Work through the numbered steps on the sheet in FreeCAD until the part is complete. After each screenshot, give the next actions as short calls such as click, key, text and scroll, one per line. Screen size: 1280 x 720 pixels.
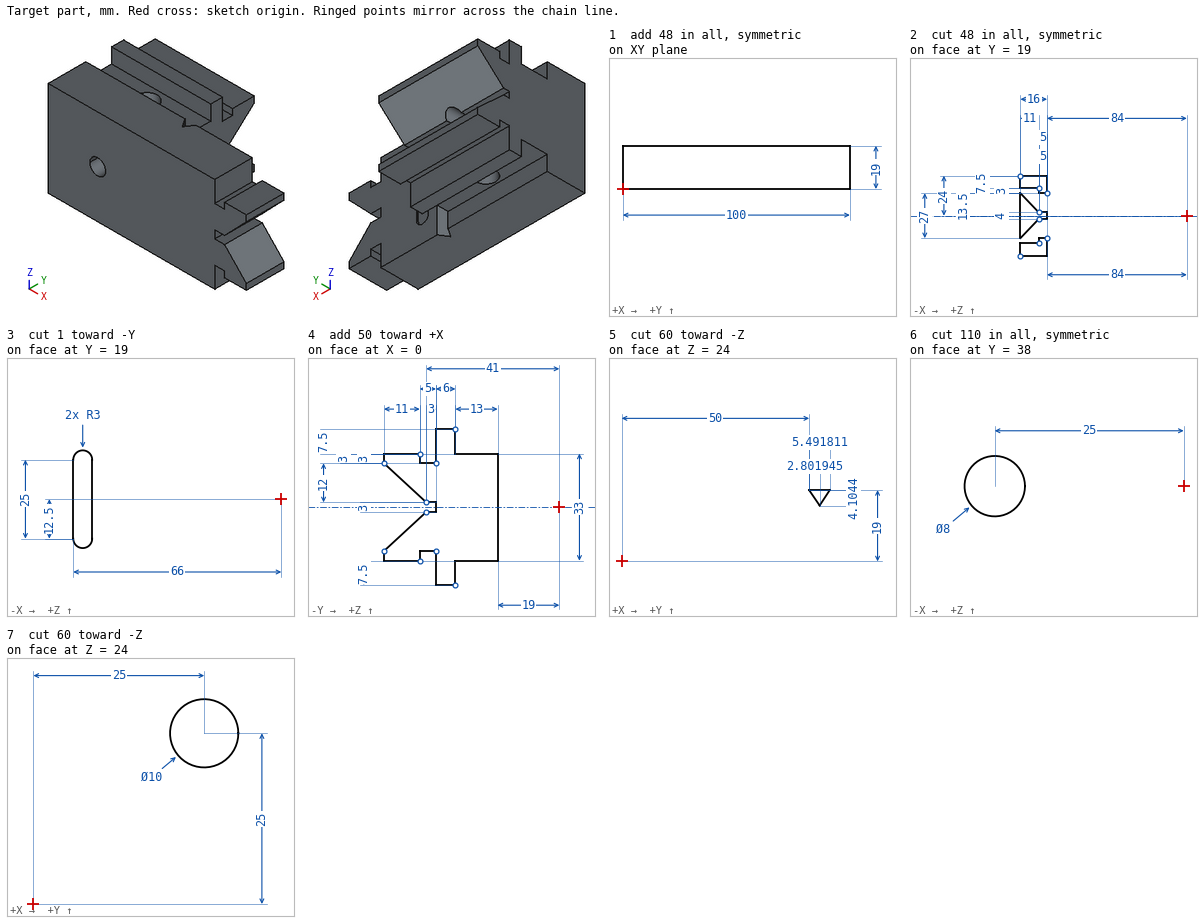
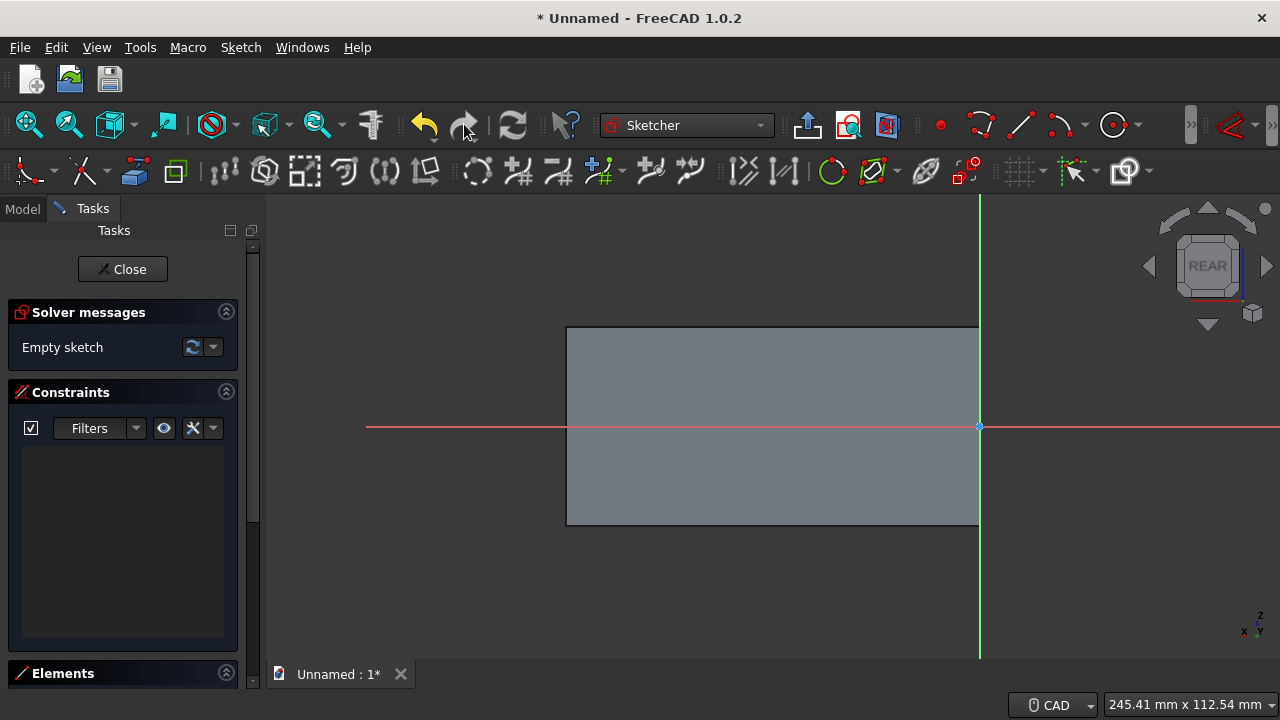
scroll(912, 426, up, 2)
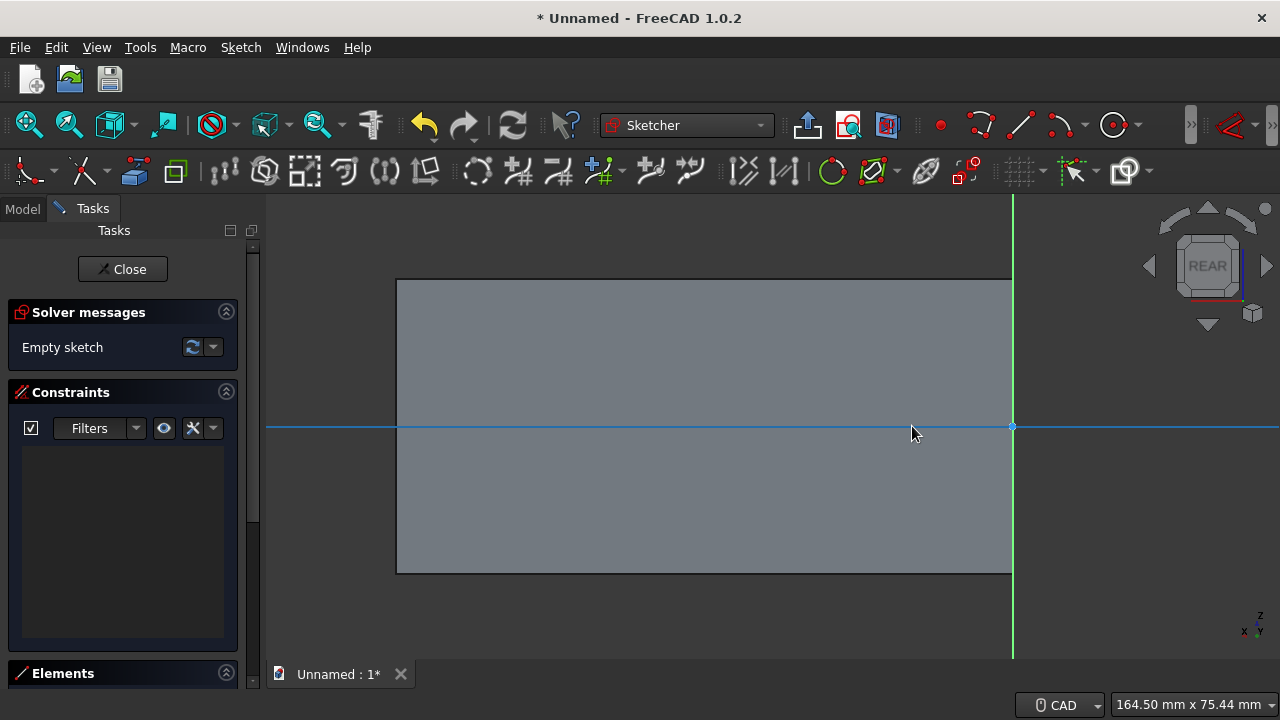
click(982, 126)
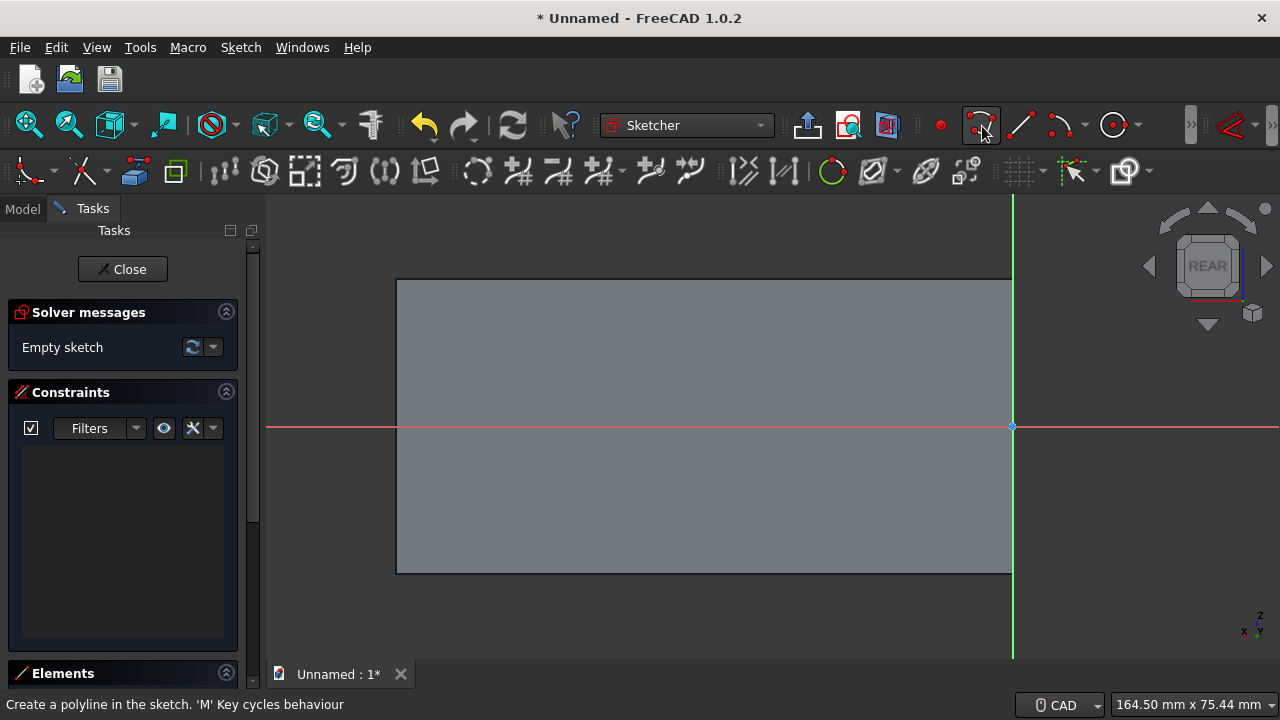
click(495, 343)
click(495, 279)
click(396, 279)
click(396, 325)
click(464, 325)
click(464, 343)
click(495, 344)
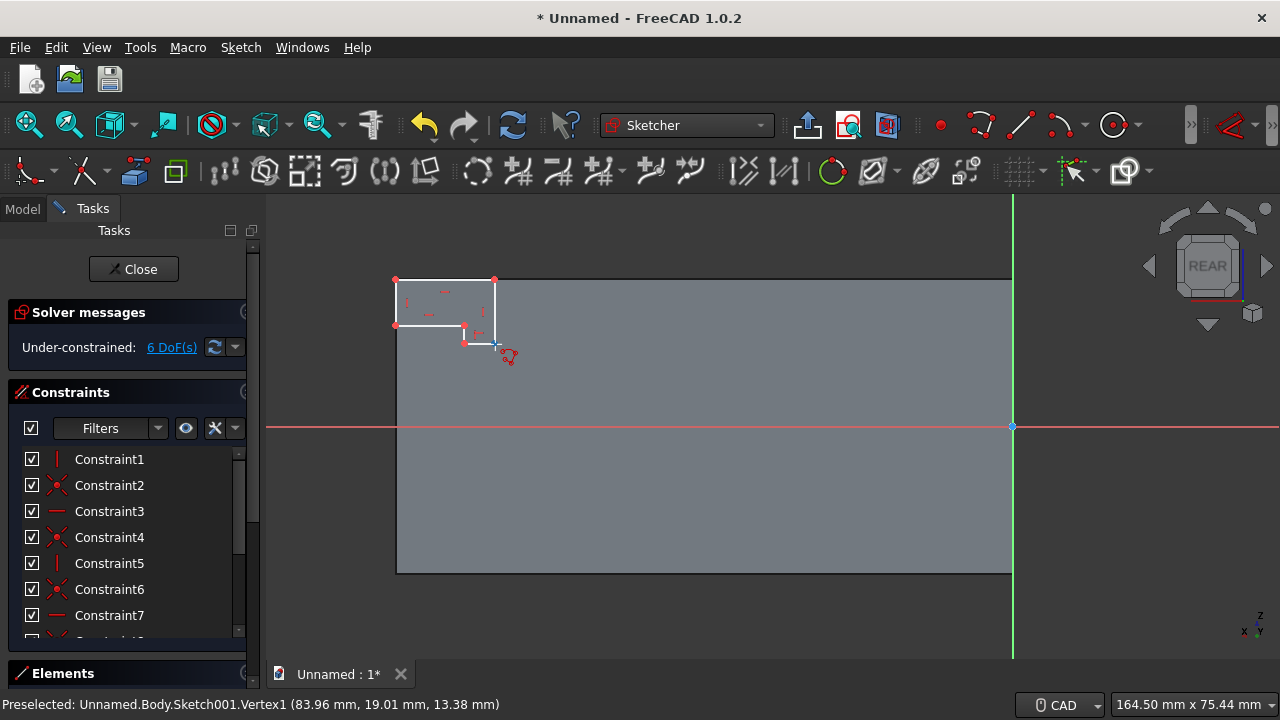
scroll(495, 439, up, 2)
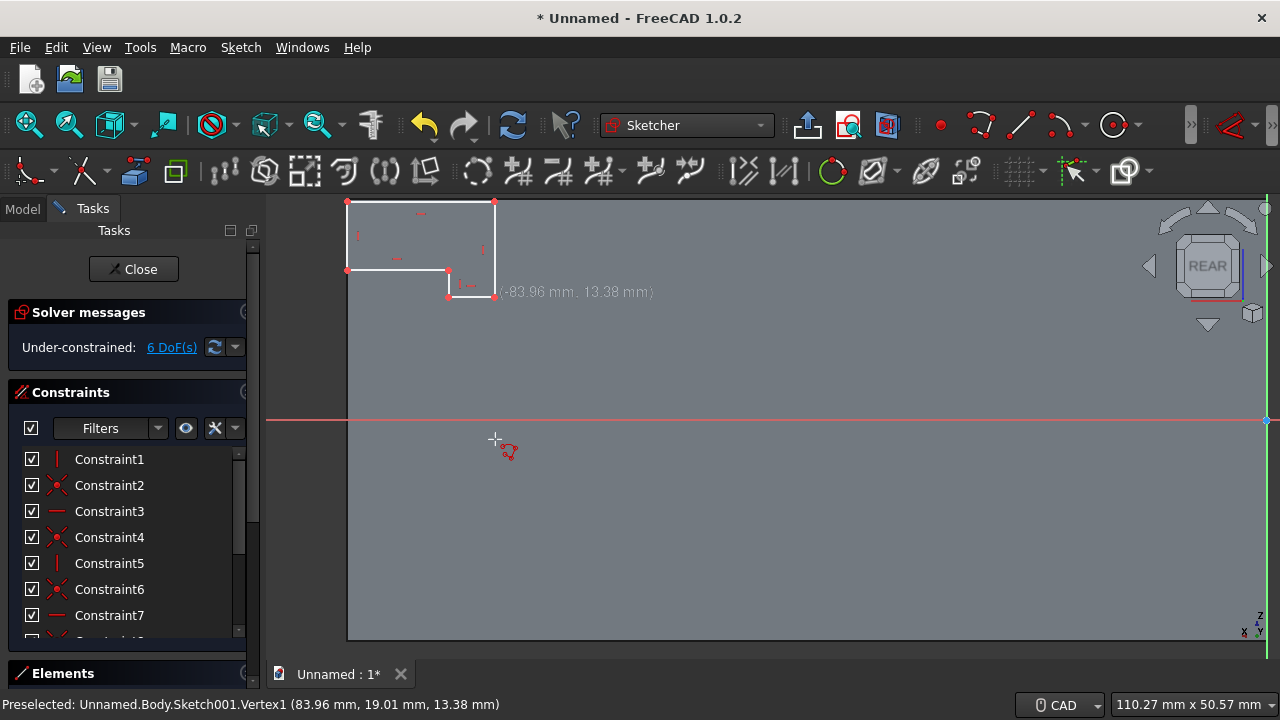
click(495, 438)
click(495, 402)
click(449, 402)
click(347, 296)
click(347, 544)
click(449, 438)
click(495, 439)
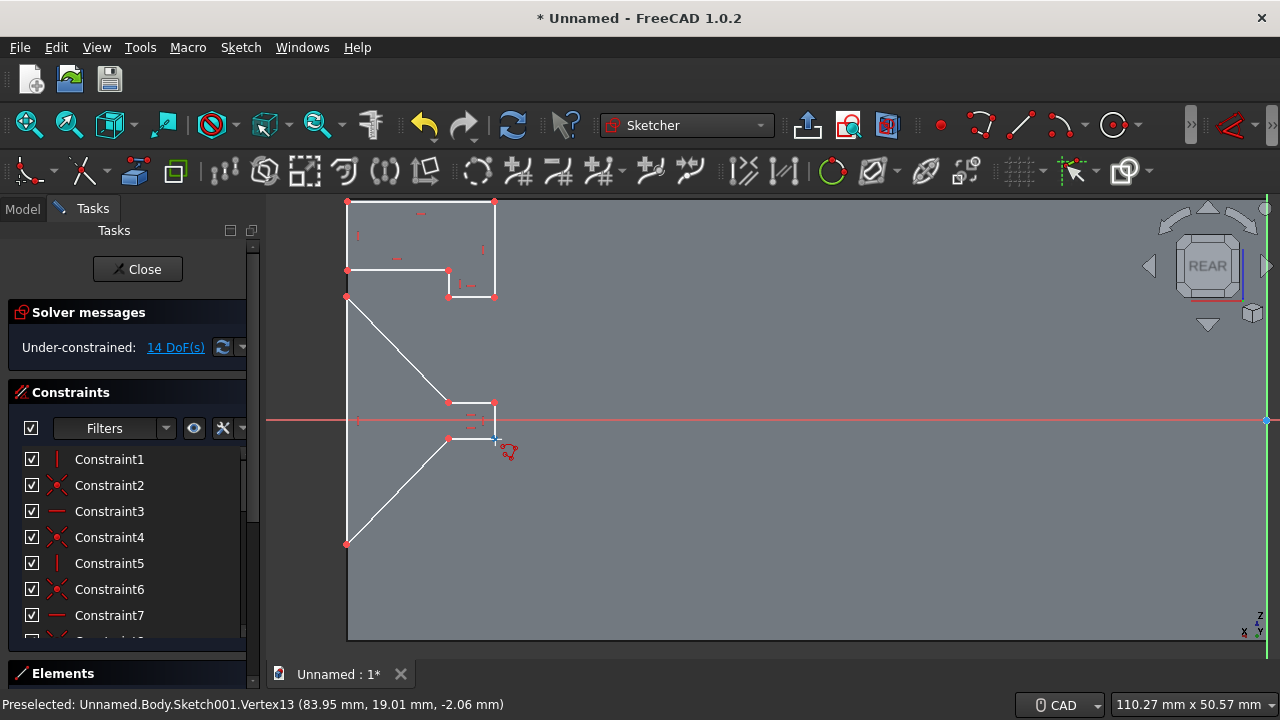
click(495, 544)
click(449, 544)
click(449, 572)
click(347, 572)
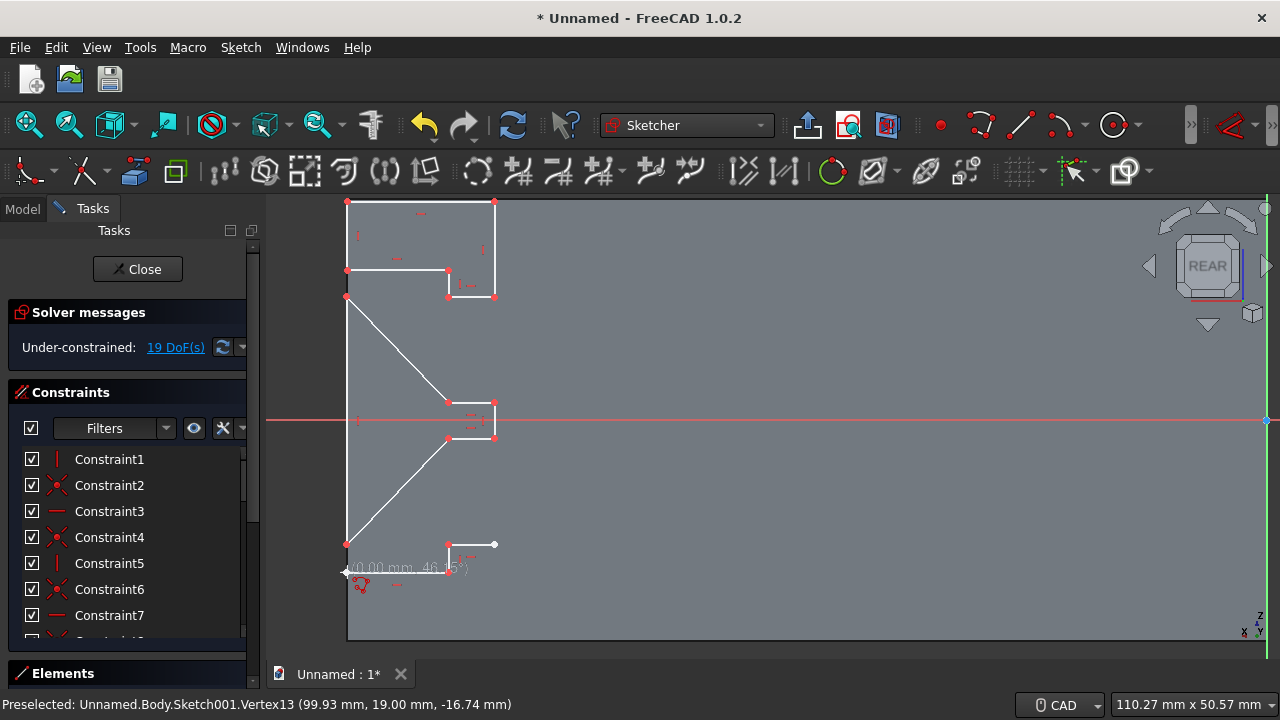
scroll(496, 440, down, 2)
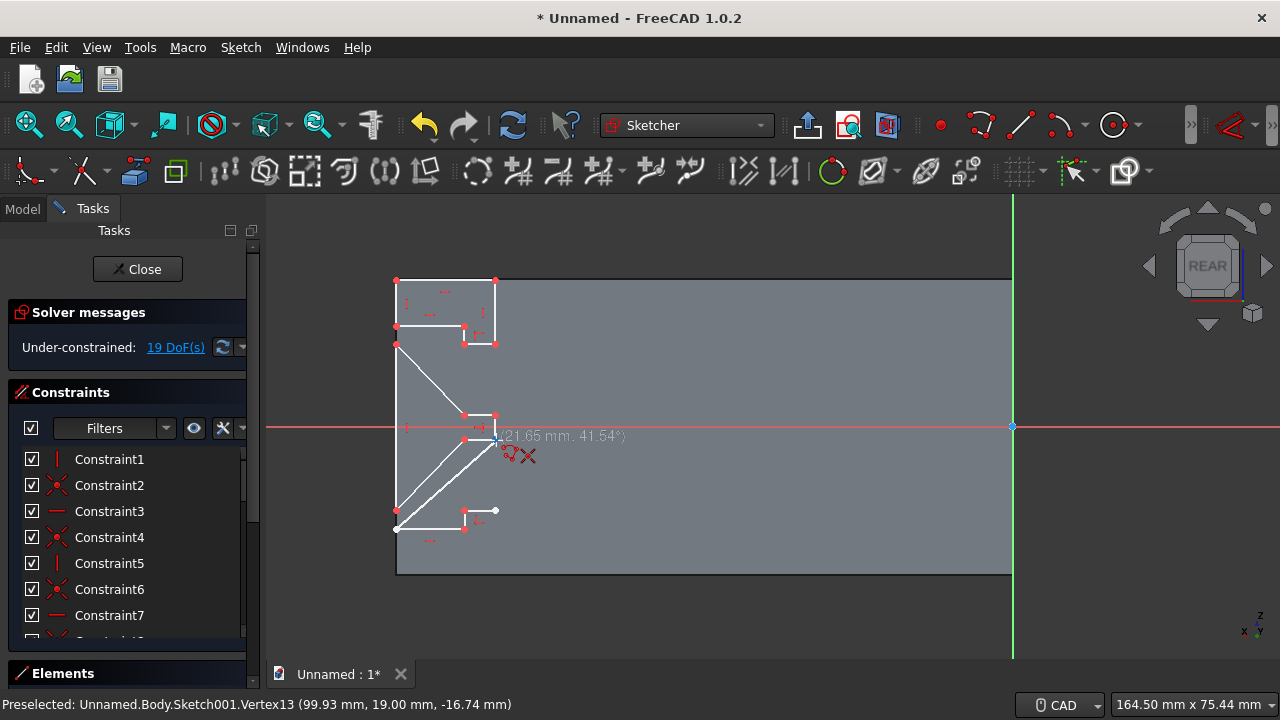
click(396, 575)
click(495, 575)
click(495, 511)
key(Escape)
key(Escape)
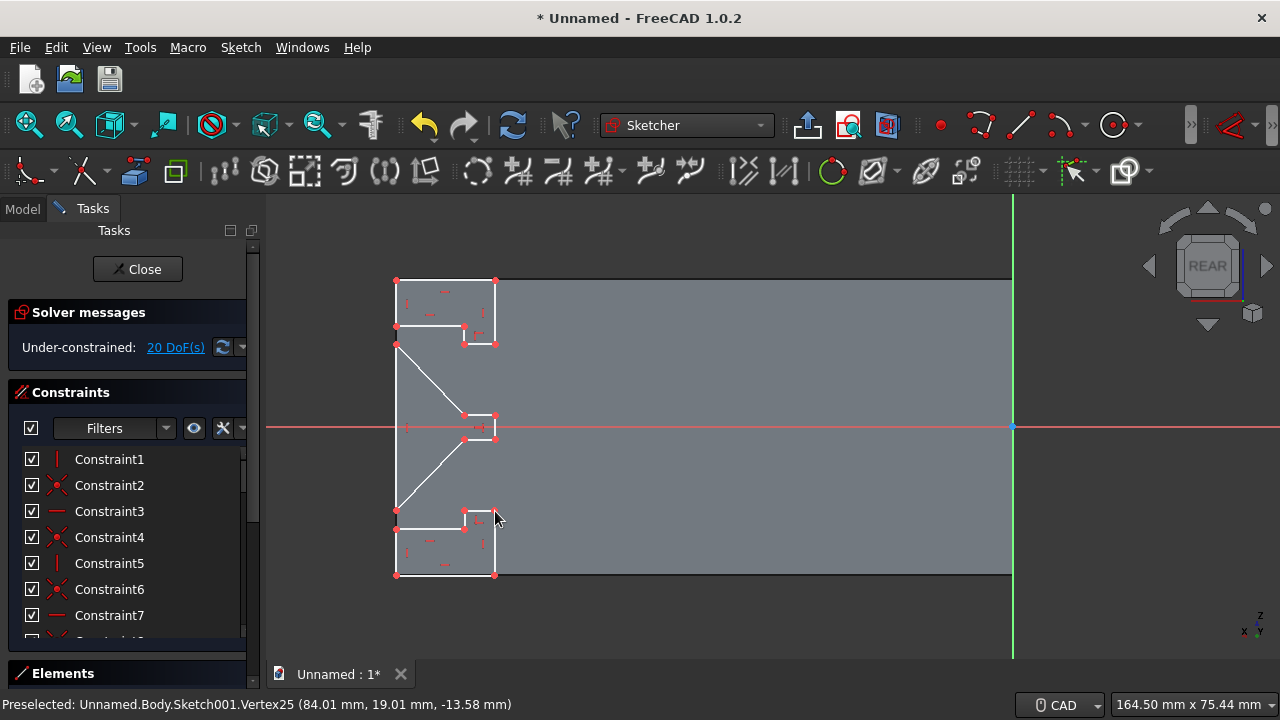
click(465, 415)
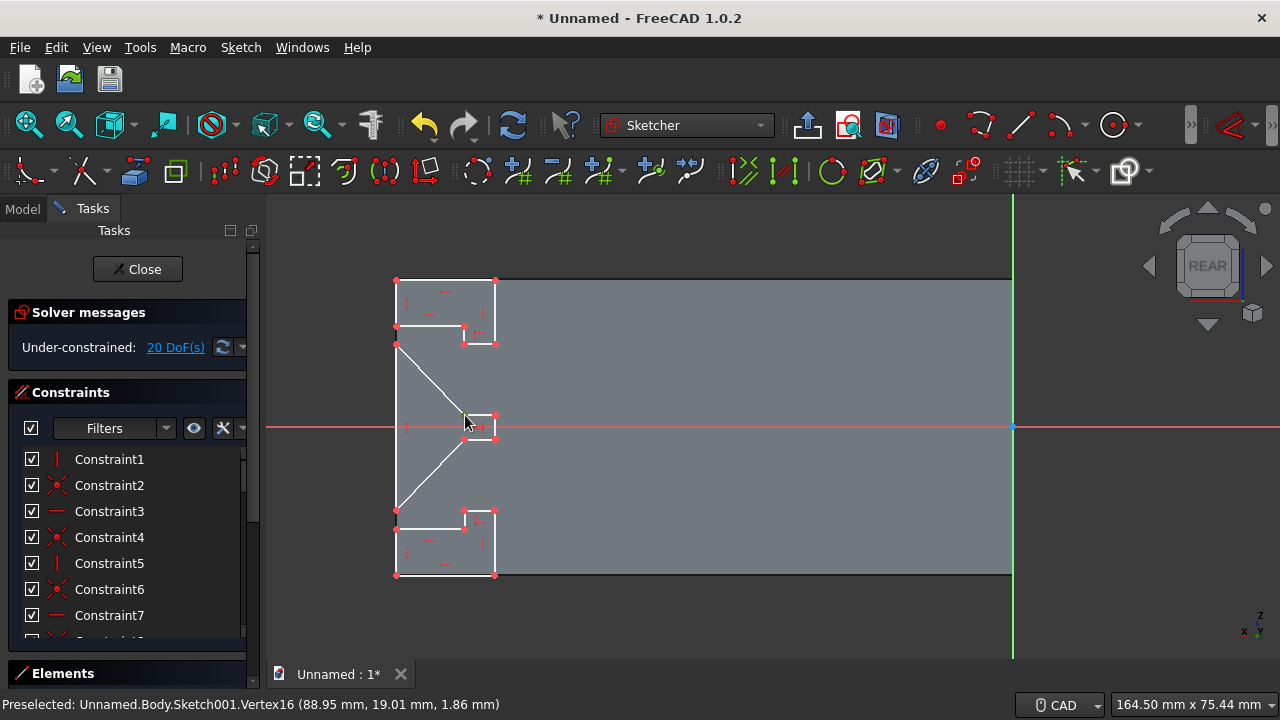
click(465, 440)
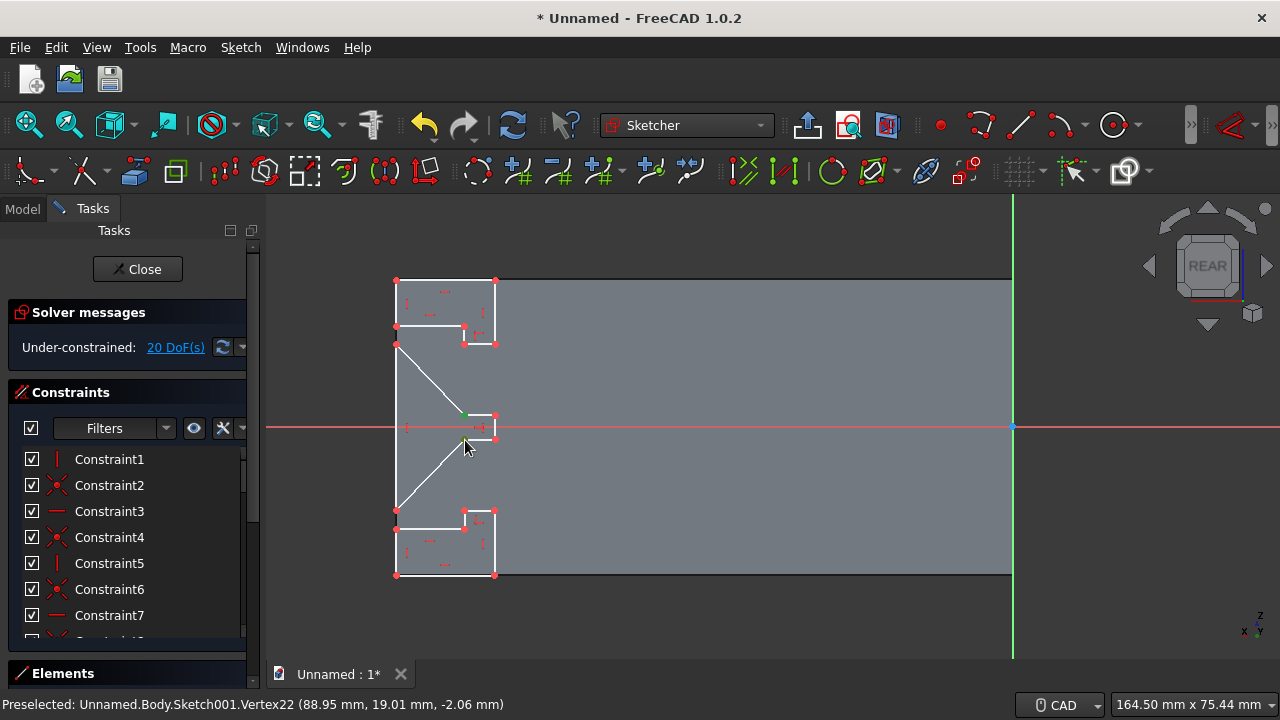
click(353, 427)